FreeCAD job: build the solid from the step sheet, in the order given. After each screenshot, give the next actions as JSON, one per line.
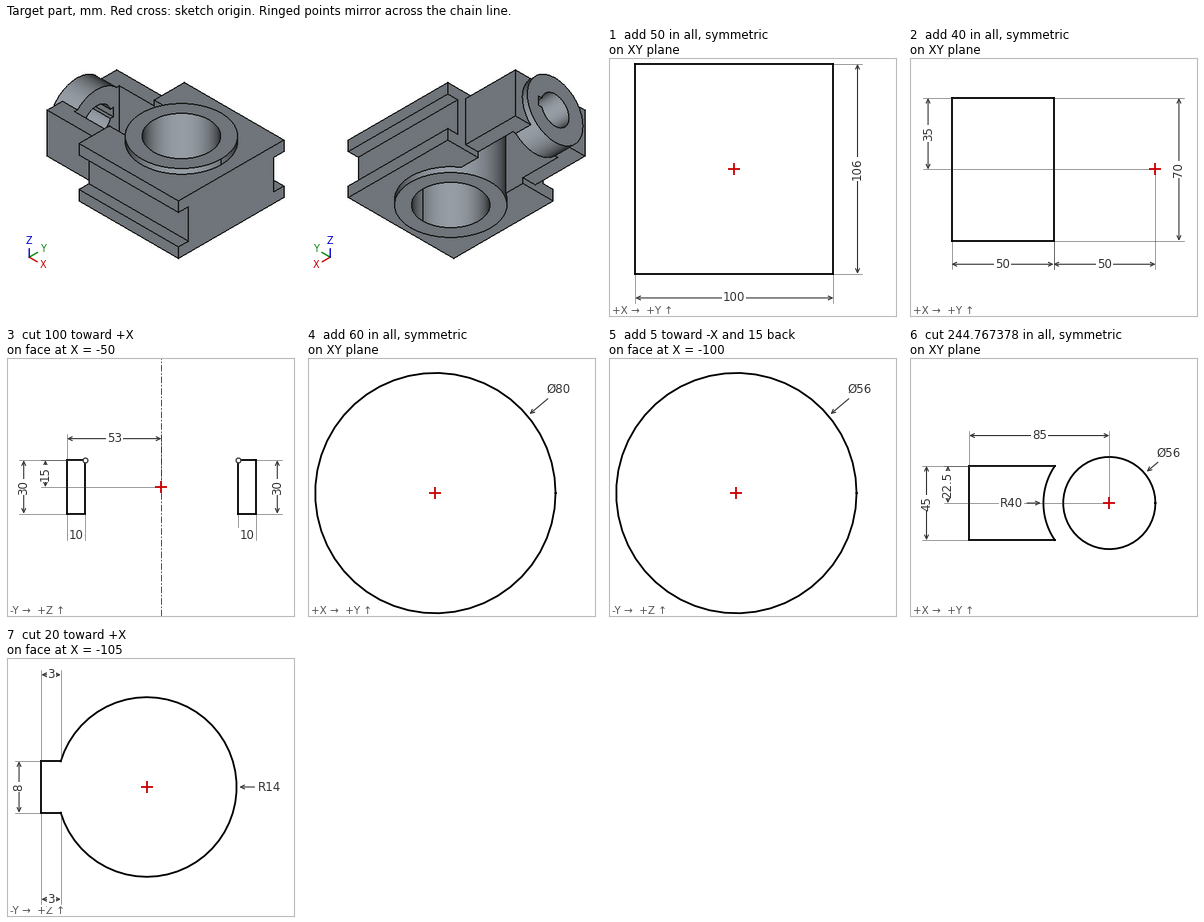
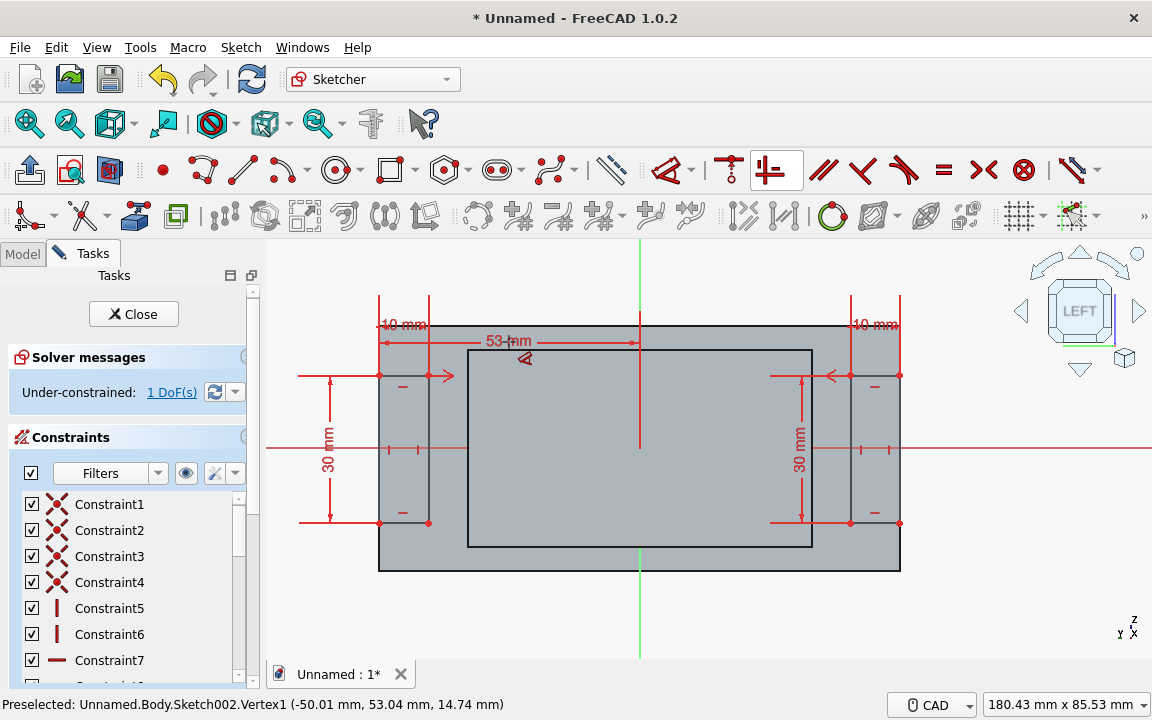
{"action": "left_click", "coordinate": [379, 376]}
{"action": "left_click", "coordinate": [345, 412]}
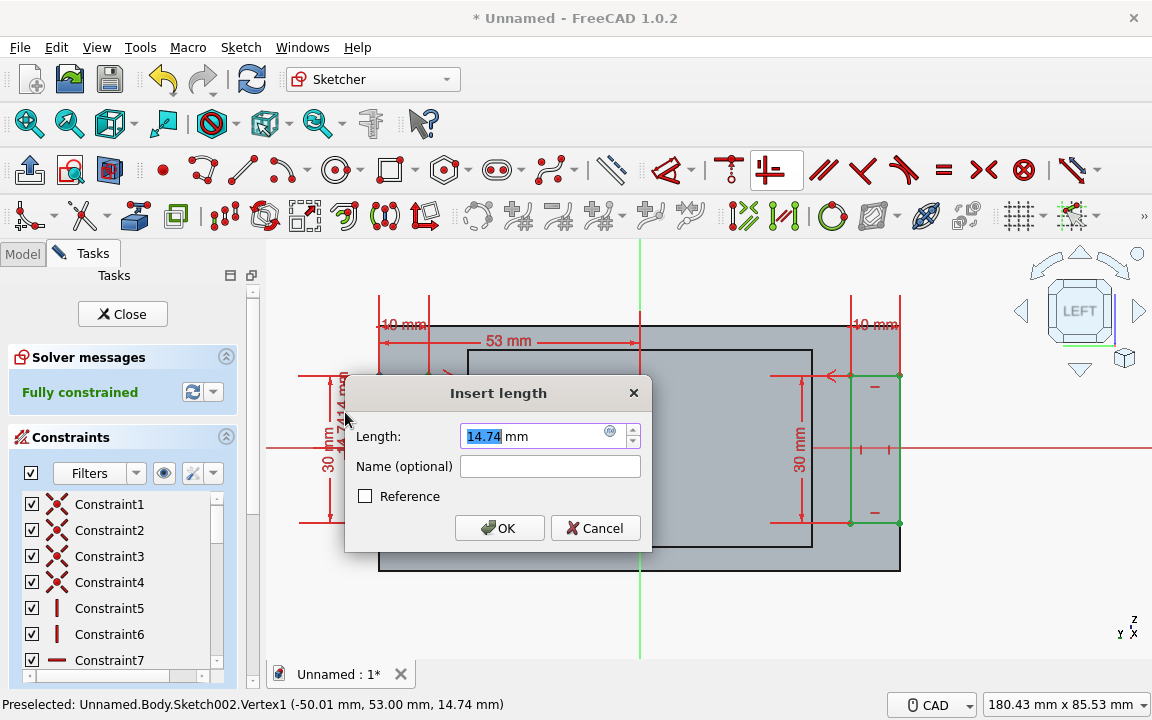
{"action": "type", "text": "15"}
{"action": "key", "text": "Return"}
{"action": "key", "text": "Escape"}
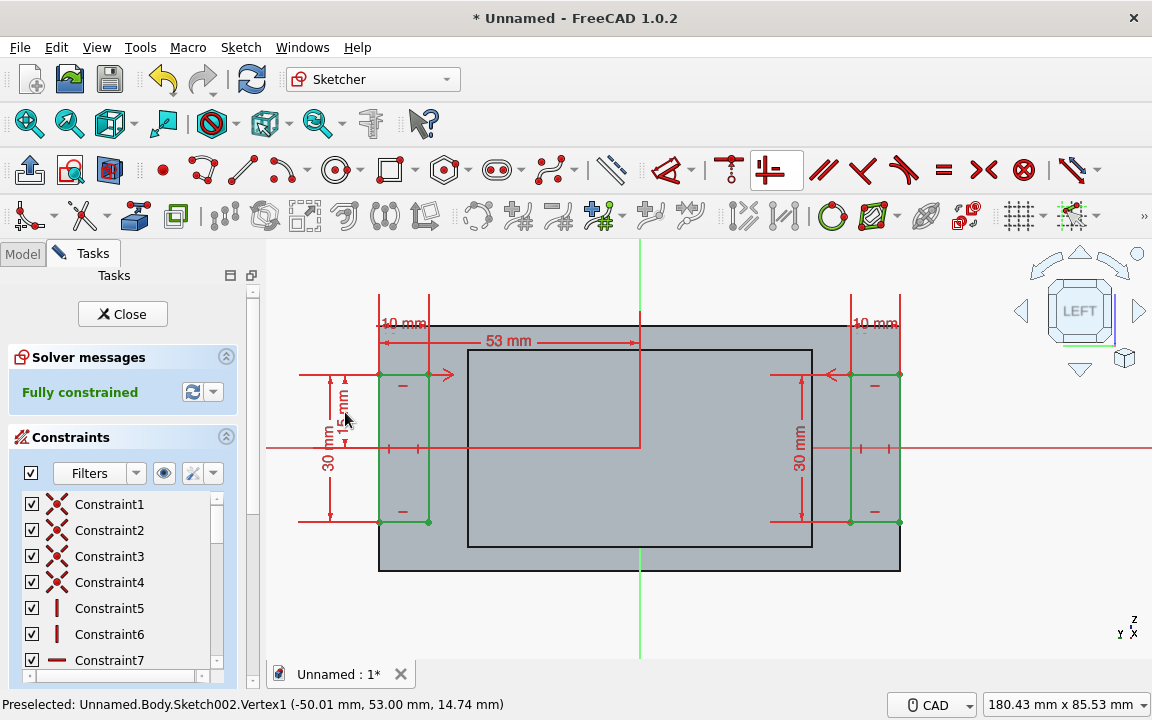
{"action": "left_click", "coordinate": [123, 314]}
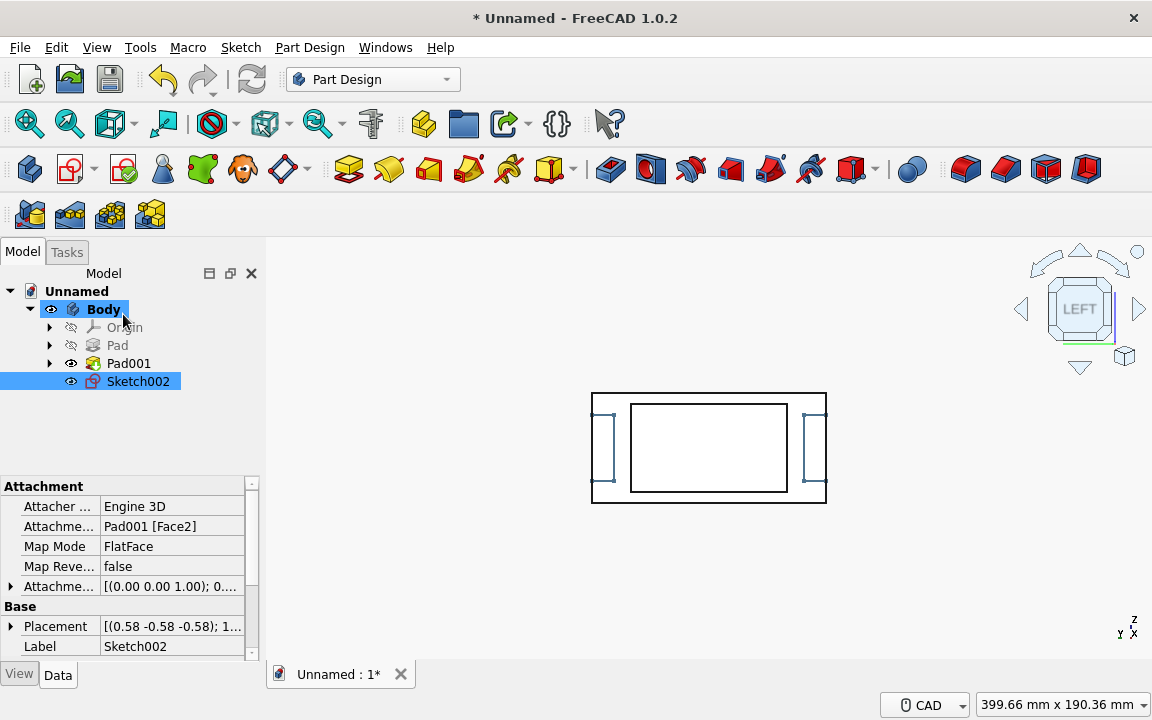
{"action": "left_click", "coordinate": [612, 170]}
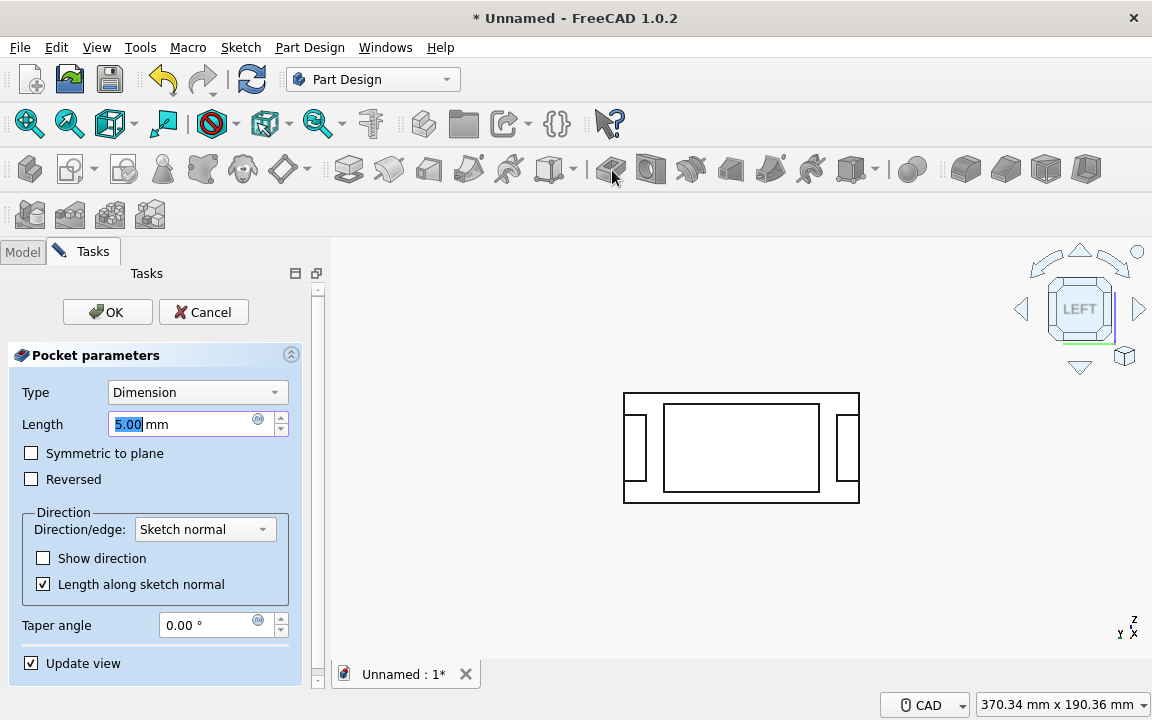
{"action": "type", "text": "100"}
{"action": "key", "text": "Tab"}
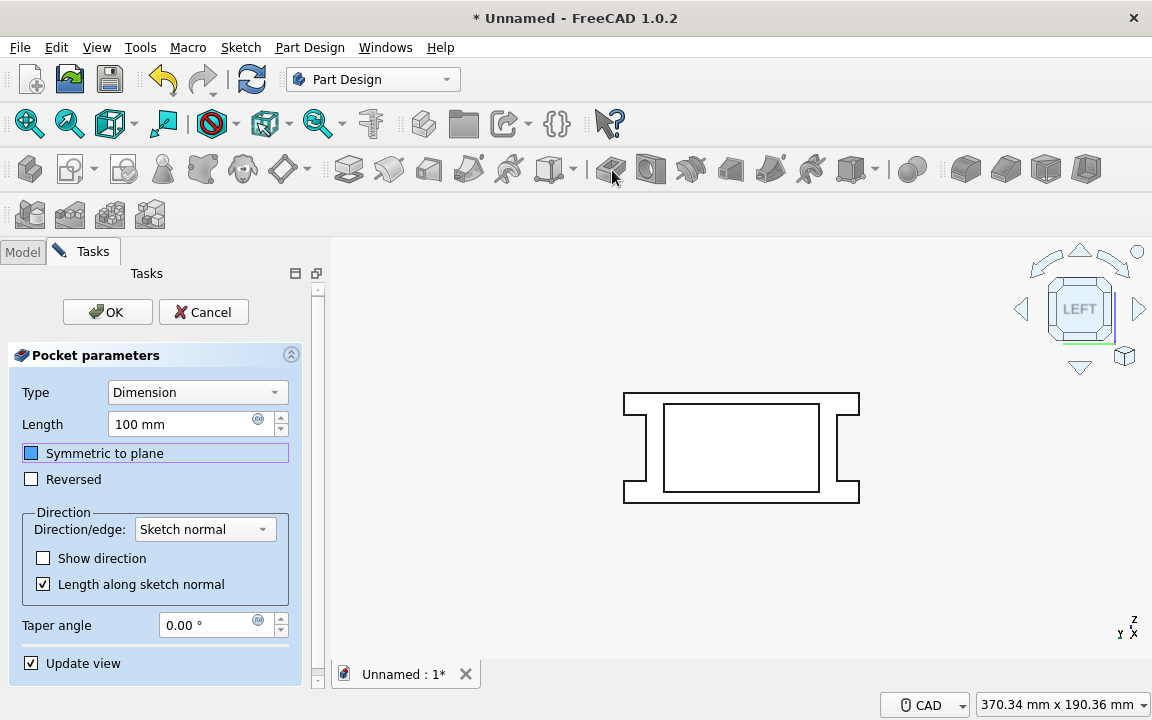
{"action": "left_click", "coordinate": [108, 312]}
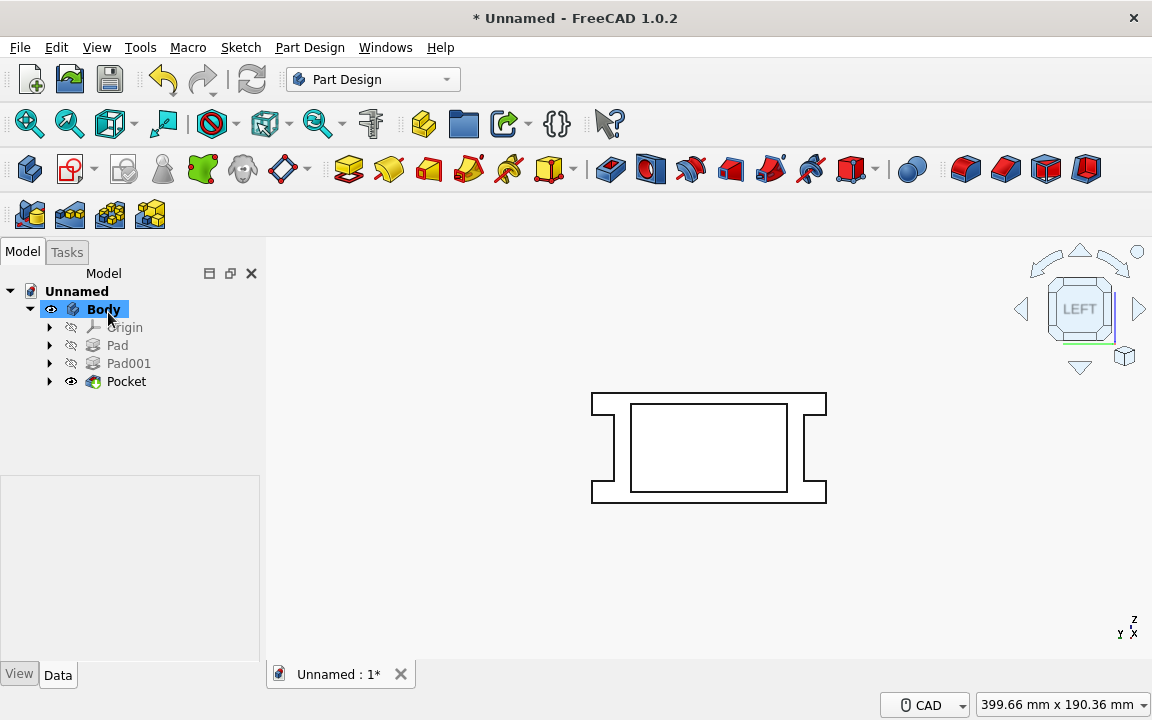
{"action": "left_click", "coordinate": [30, 124]}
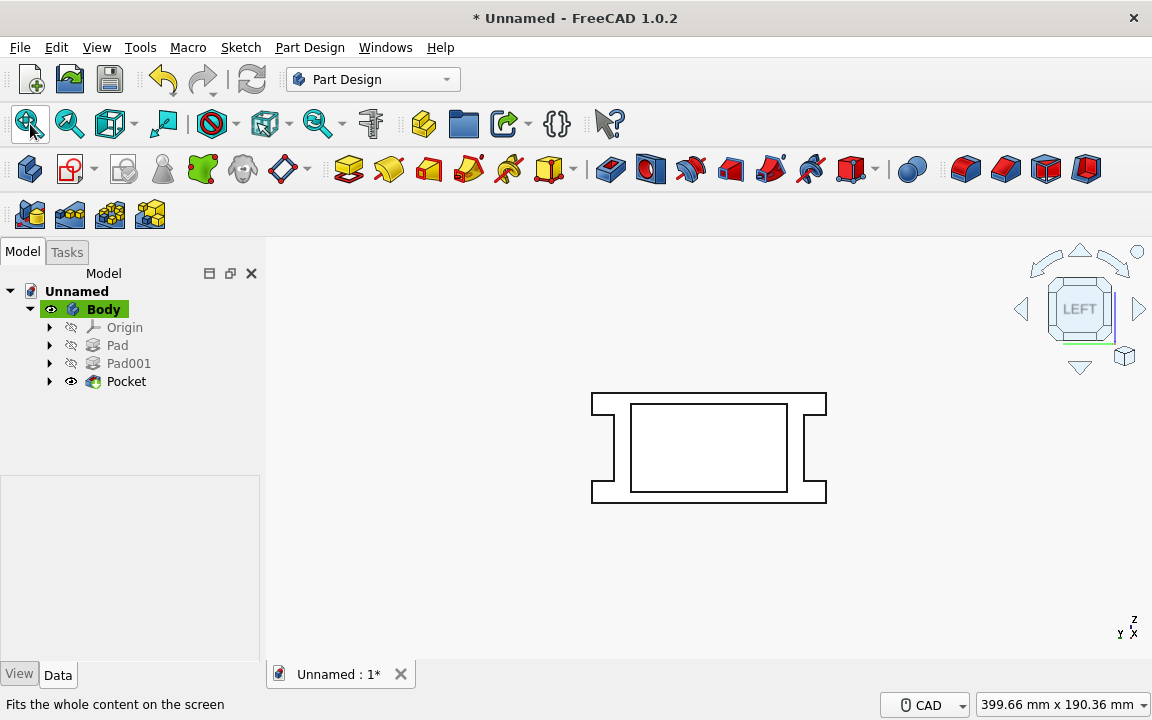
{"action": "left_click", "coordinate": [70, 170]}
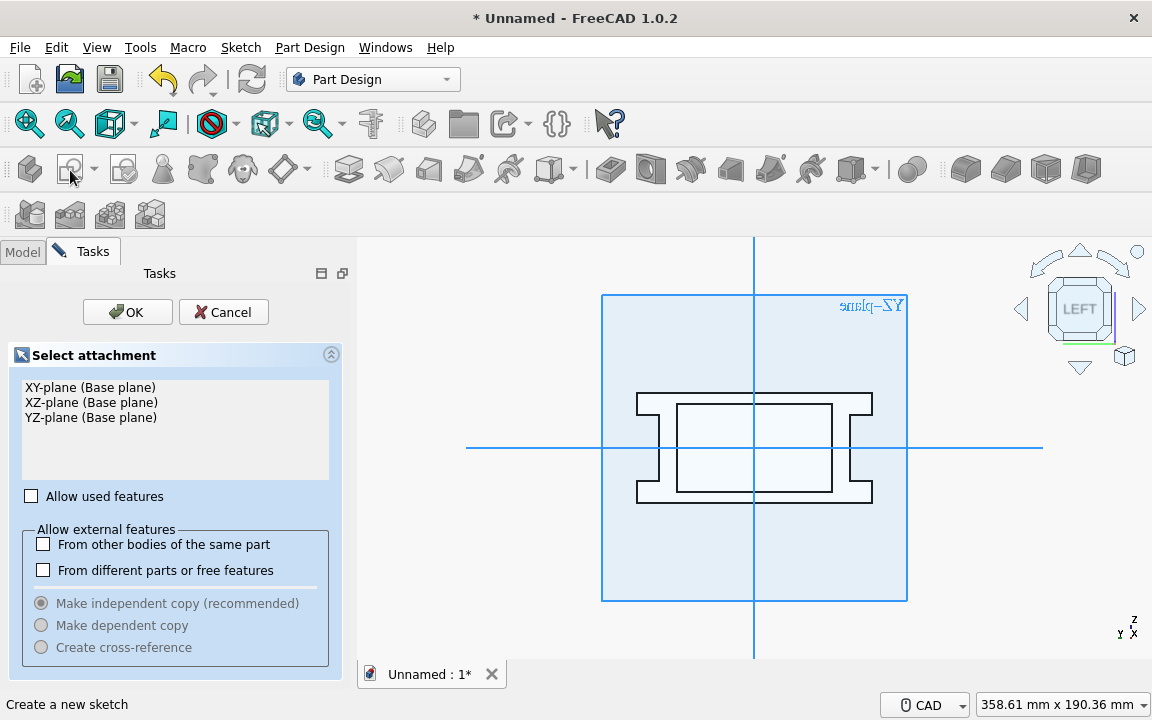
{"action": "left_click", "coordinate": [82, 388]}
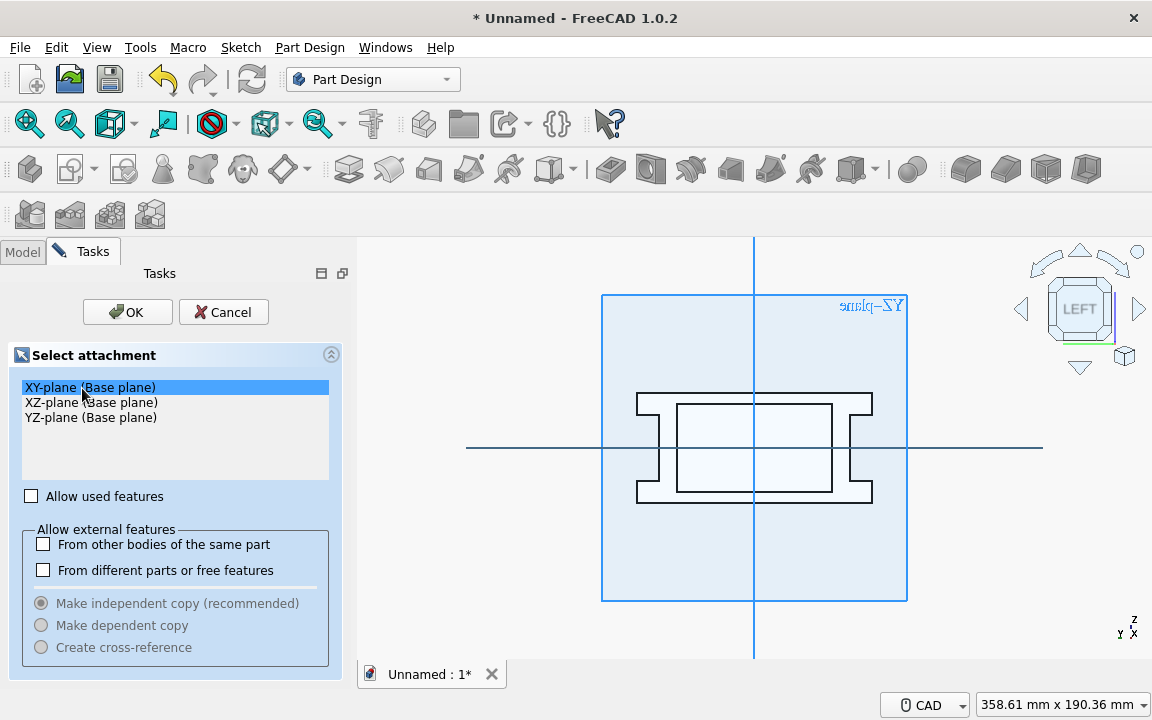
{"action": "left_click", "coordinate": [128, 312]}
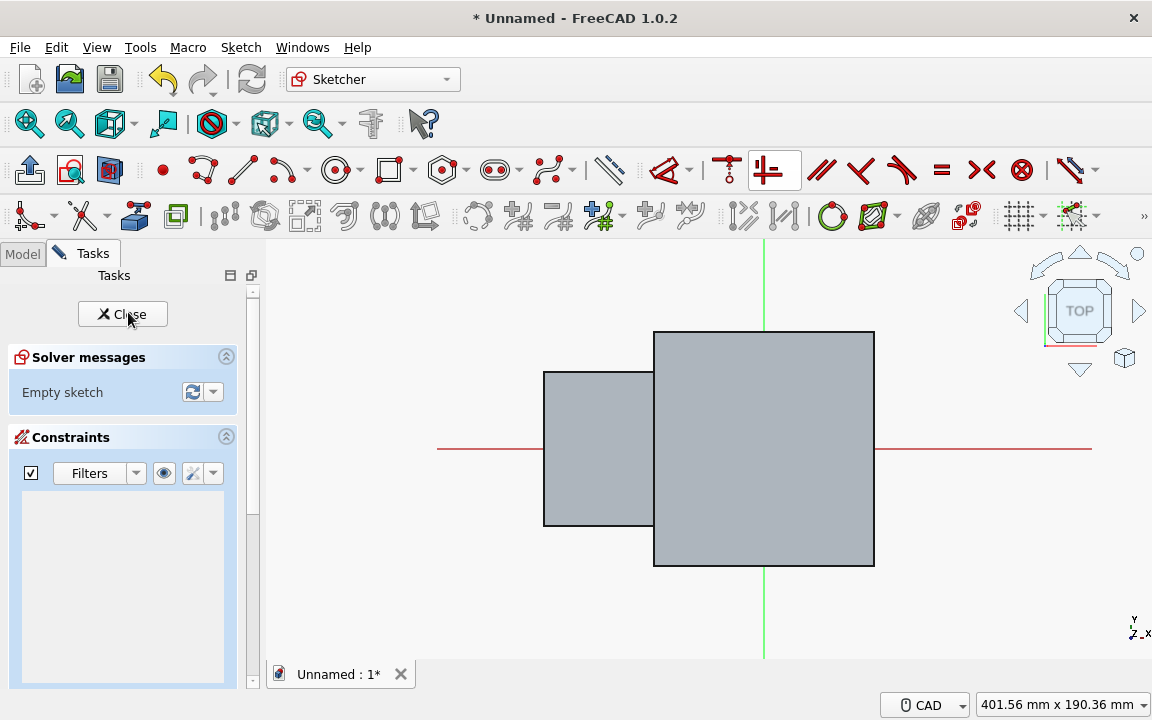
{"action": "left_click", "coordinate": [110, 170]}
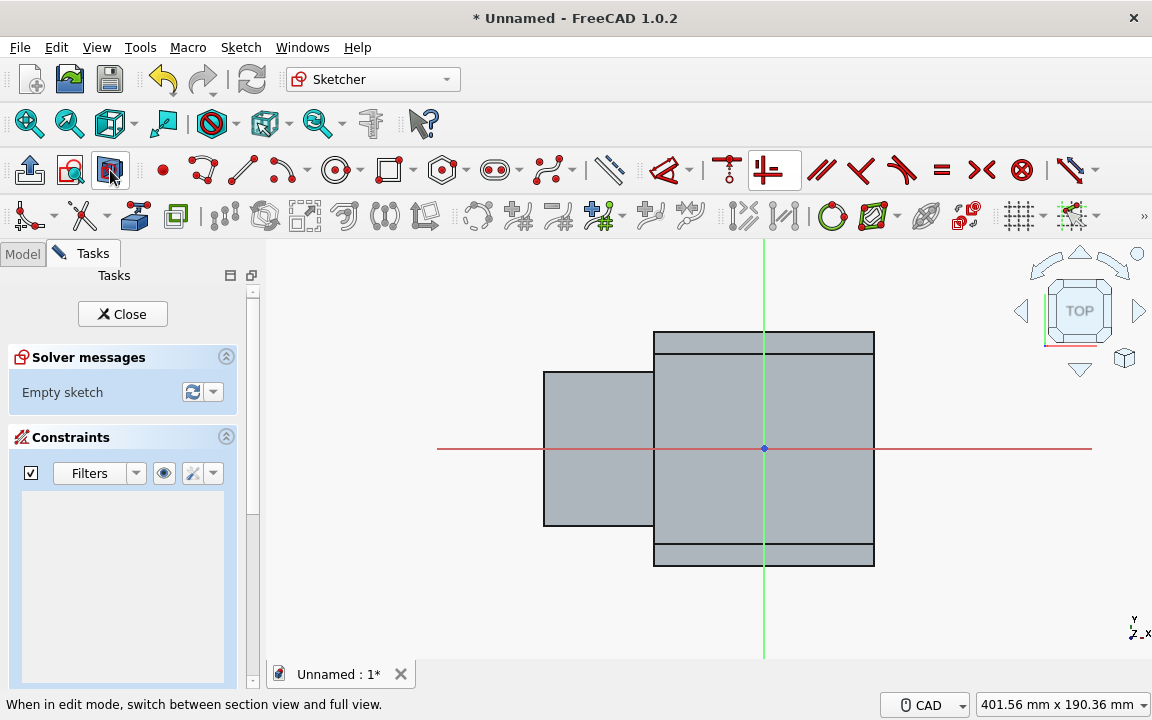
{"action": "scroll", "coordinate": [987, 449], "scroll_direction": "up", "scroll_amount": 2}